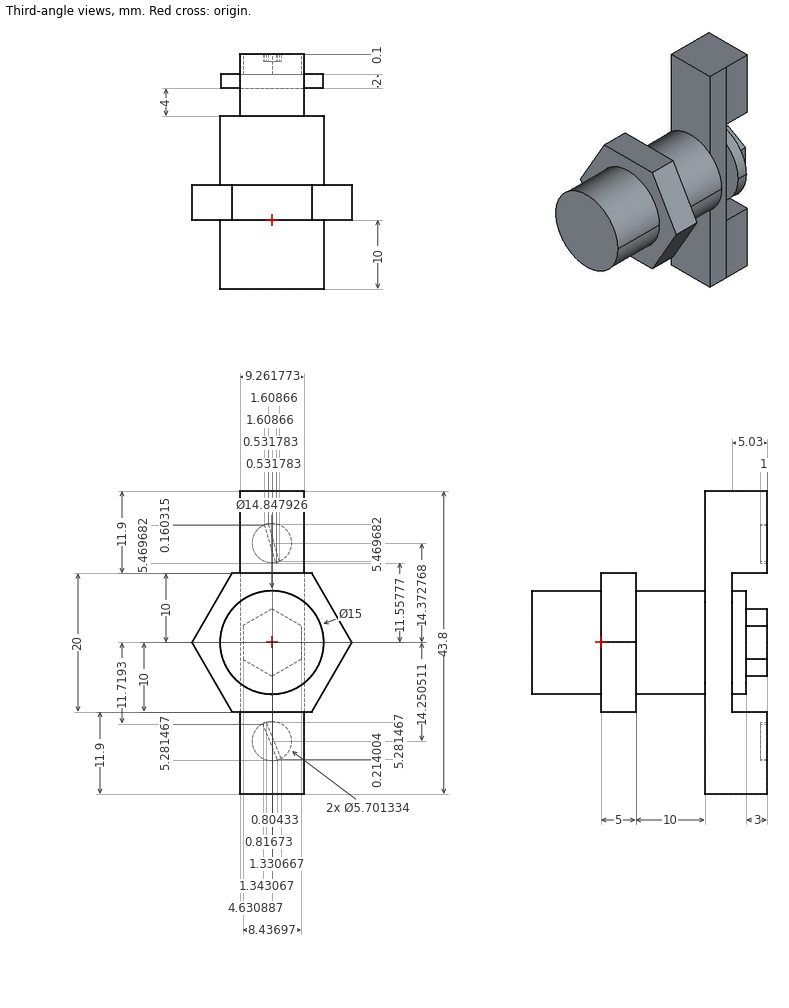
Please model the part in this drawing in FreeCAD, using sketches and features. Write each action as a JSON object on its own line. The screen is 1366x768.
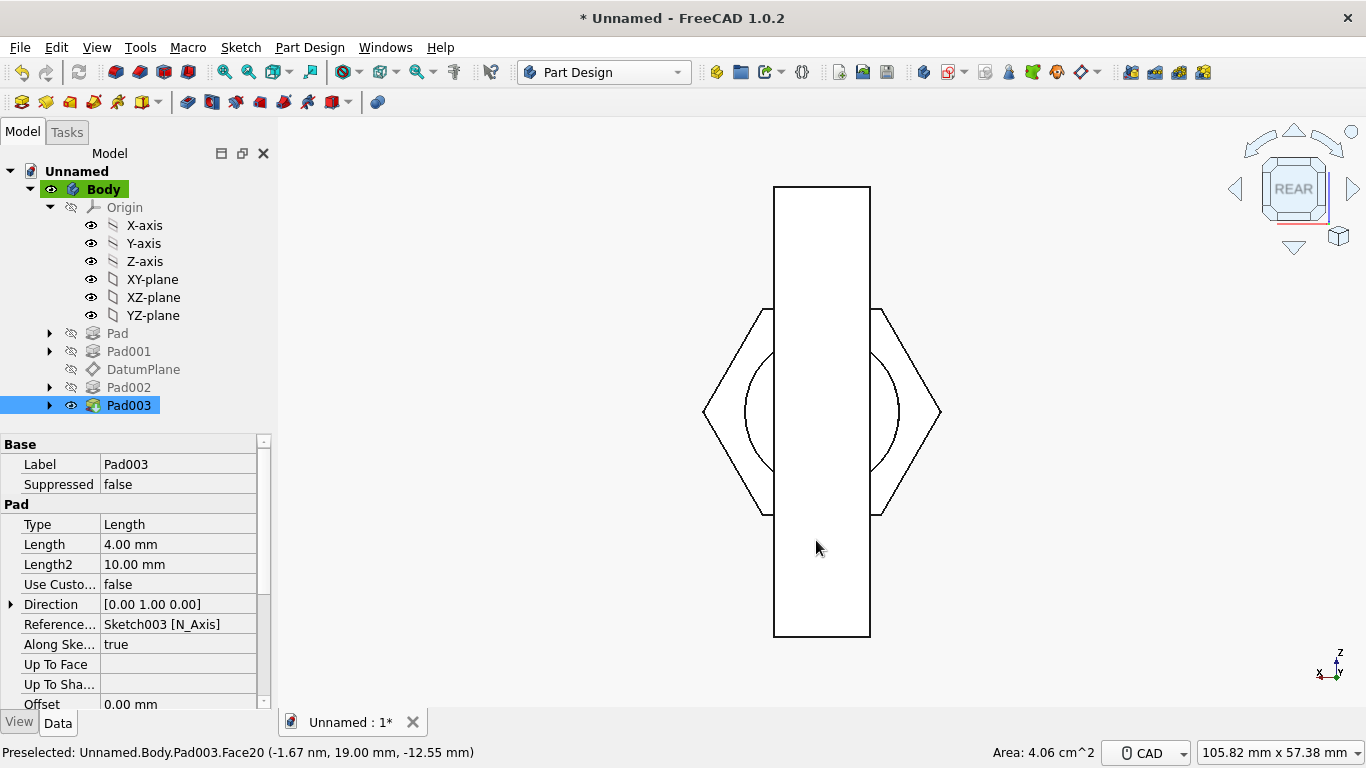
{"action": "left_click", "coordinate": [948, 72]}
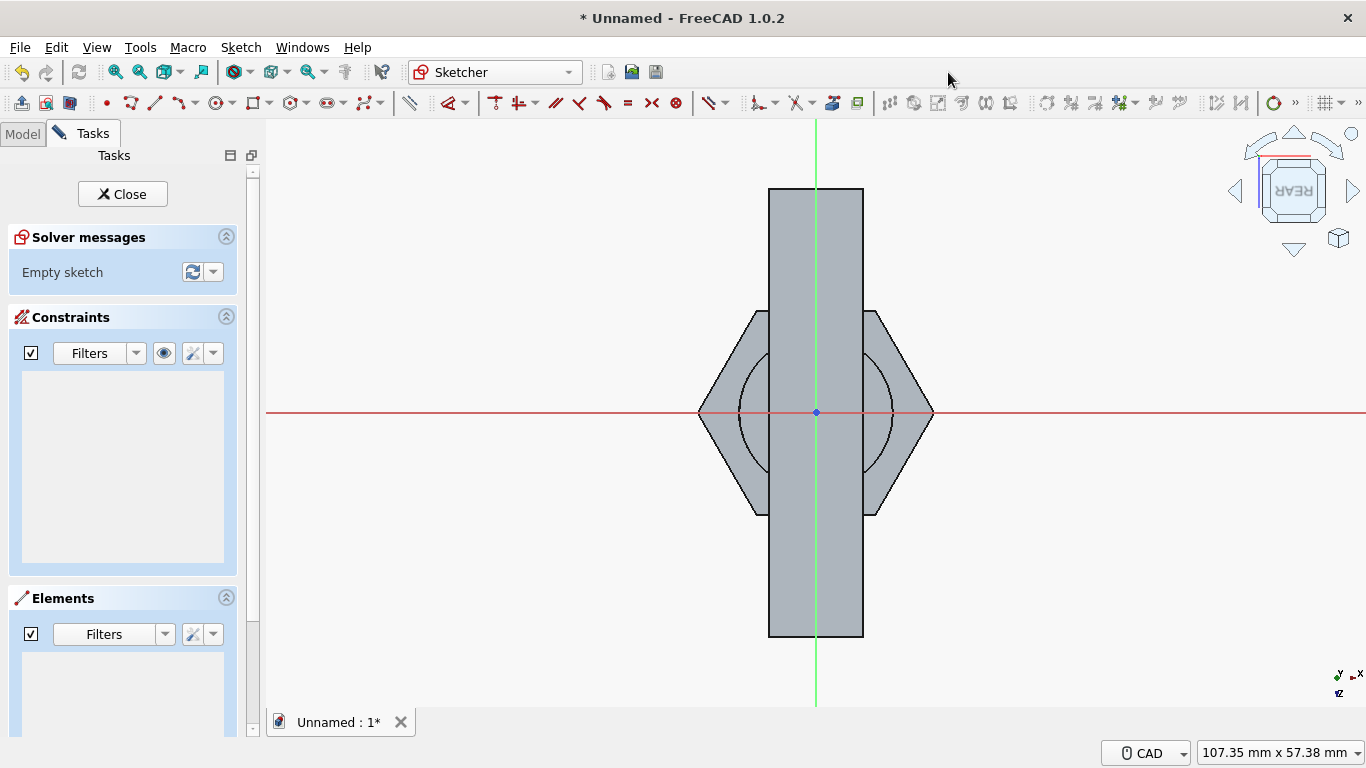
{"action": "left_click", "coordinate": [254, 104]}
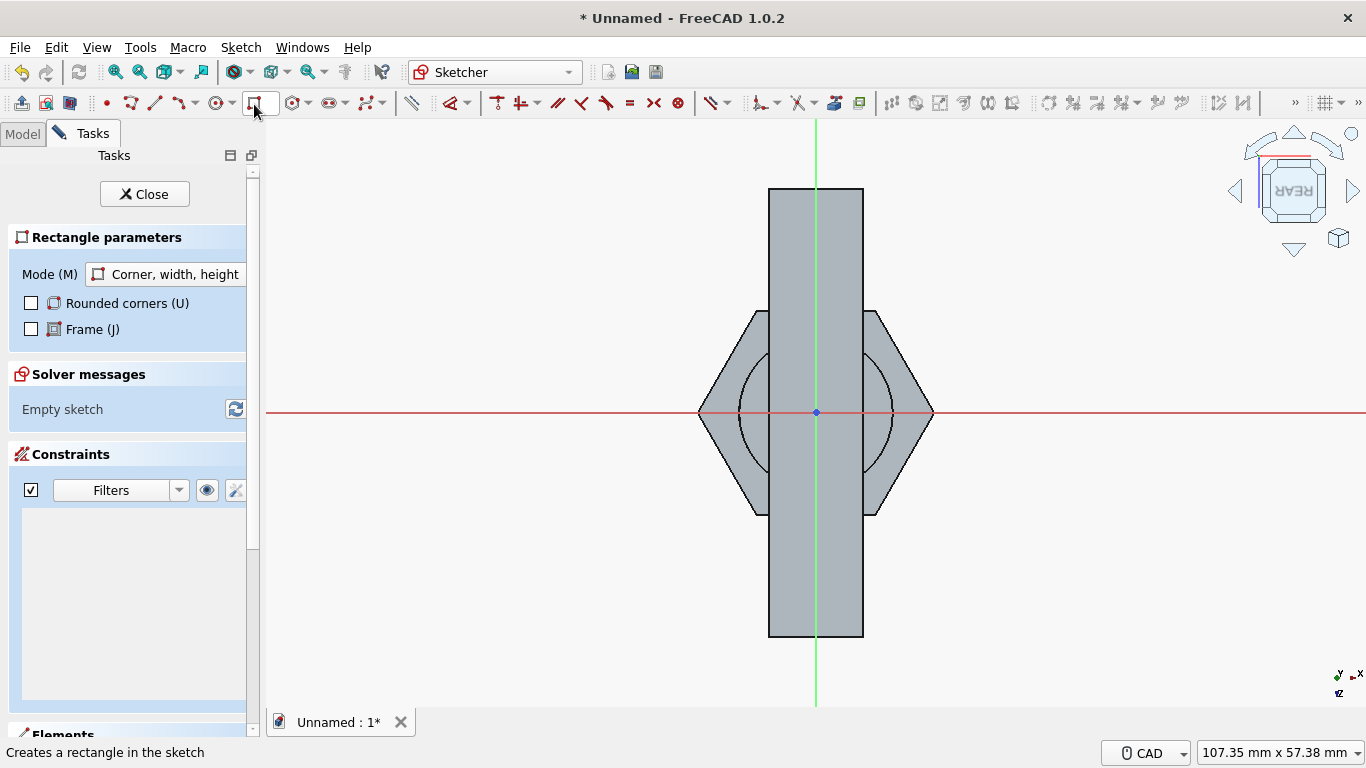
{"action": "left_click", "coordinate": [769, 189]}
{"action": "left_click", "coordinate": [863, 311]}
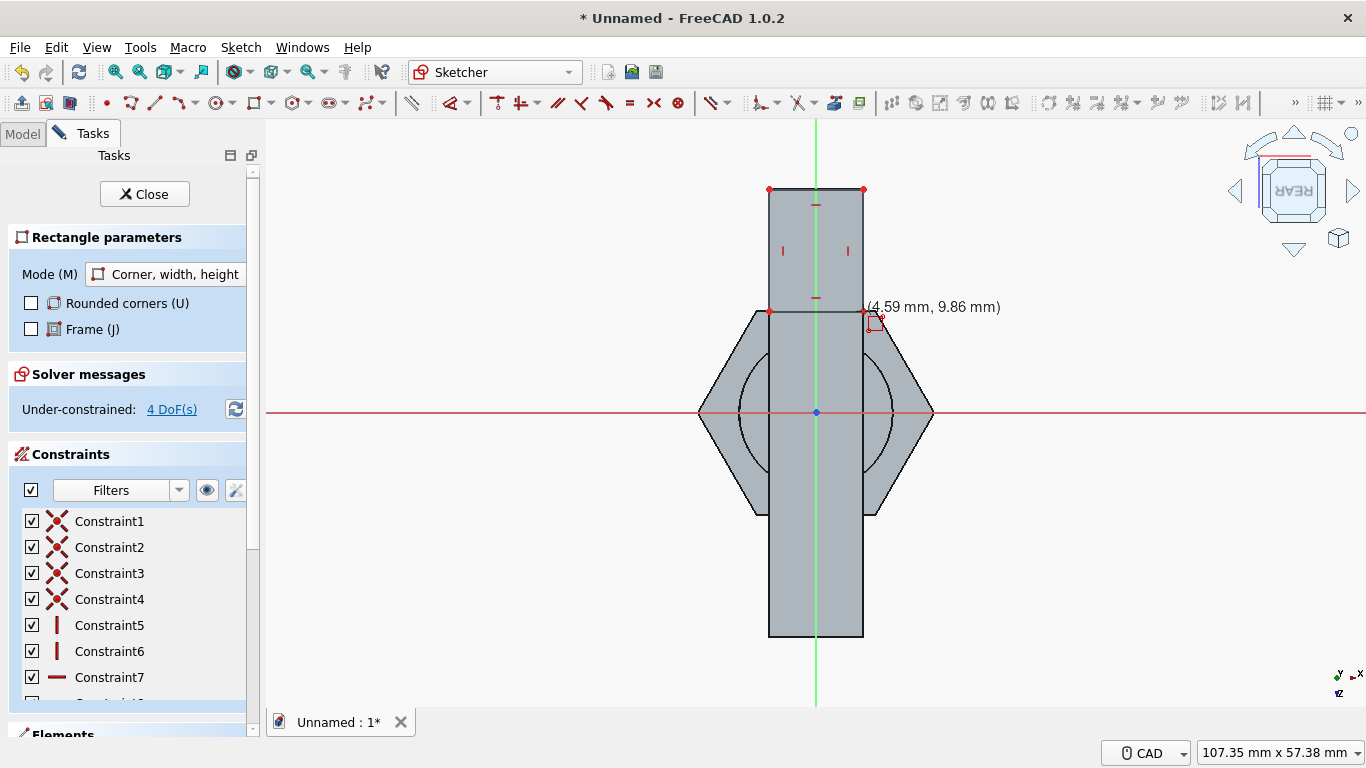
{"action": "left_click", "coordinate": [769, 515]}
{"action": "left_click", "coordinate": [863, 637]}
{"action": "key", "text": "Escape"}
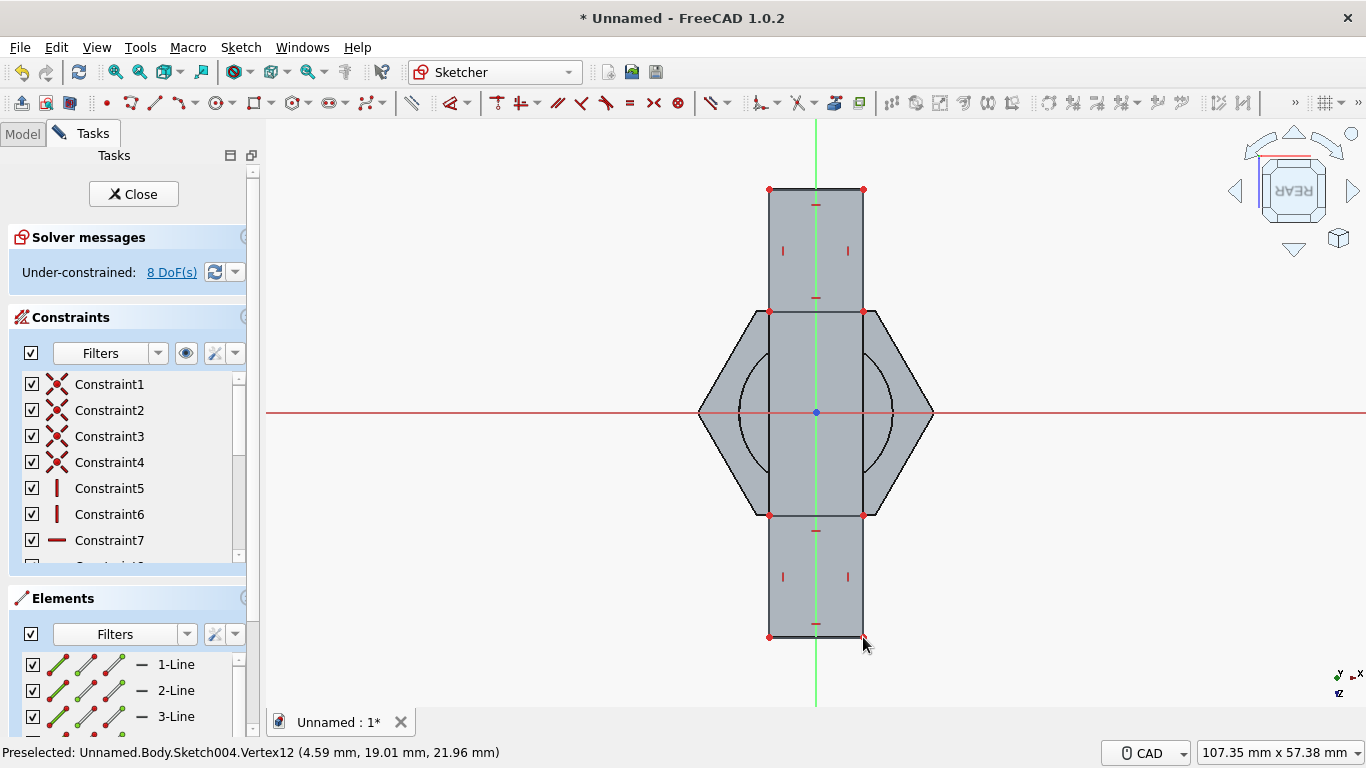
{"action": "left_click", "coordinate": [450, 104]}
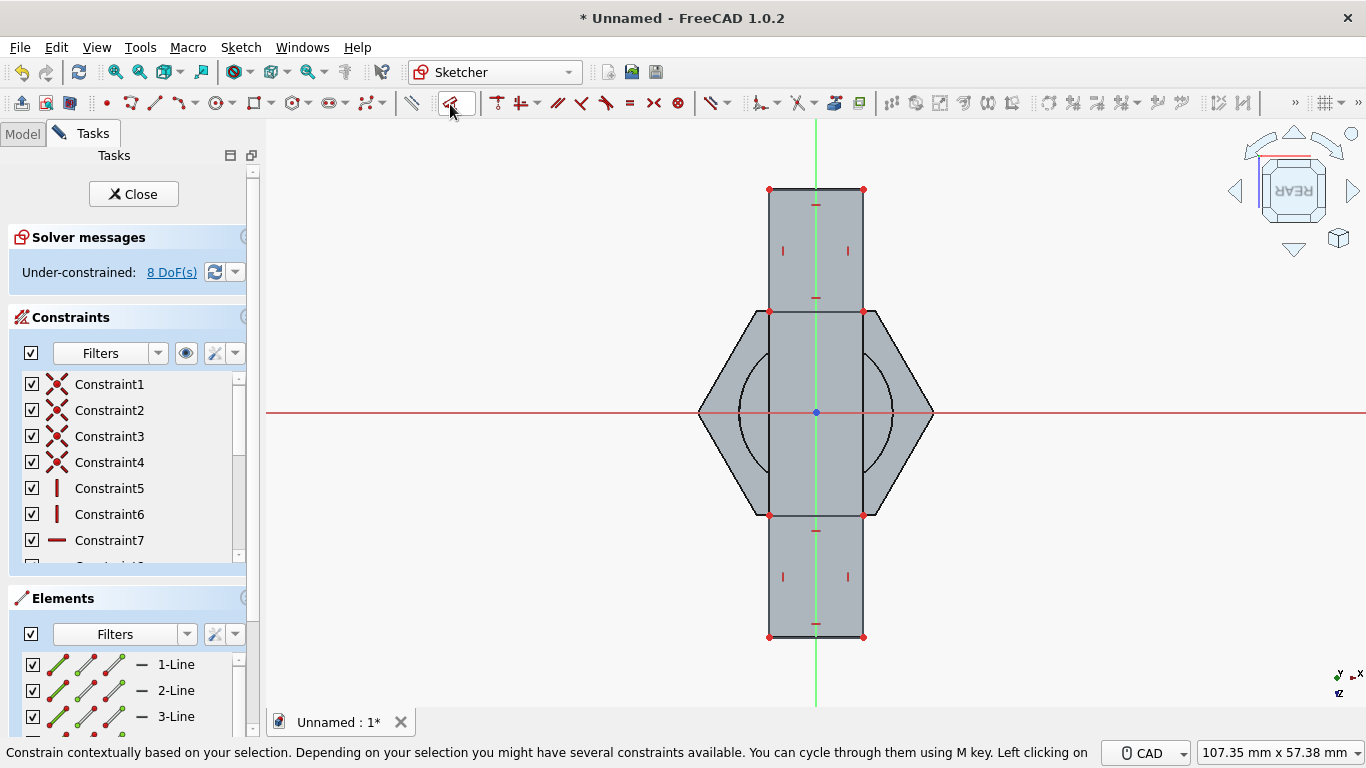
{"action": "left_click", "coordinate": [769, 312]}
{"action": "left_click", "coordinate": [735, 362]}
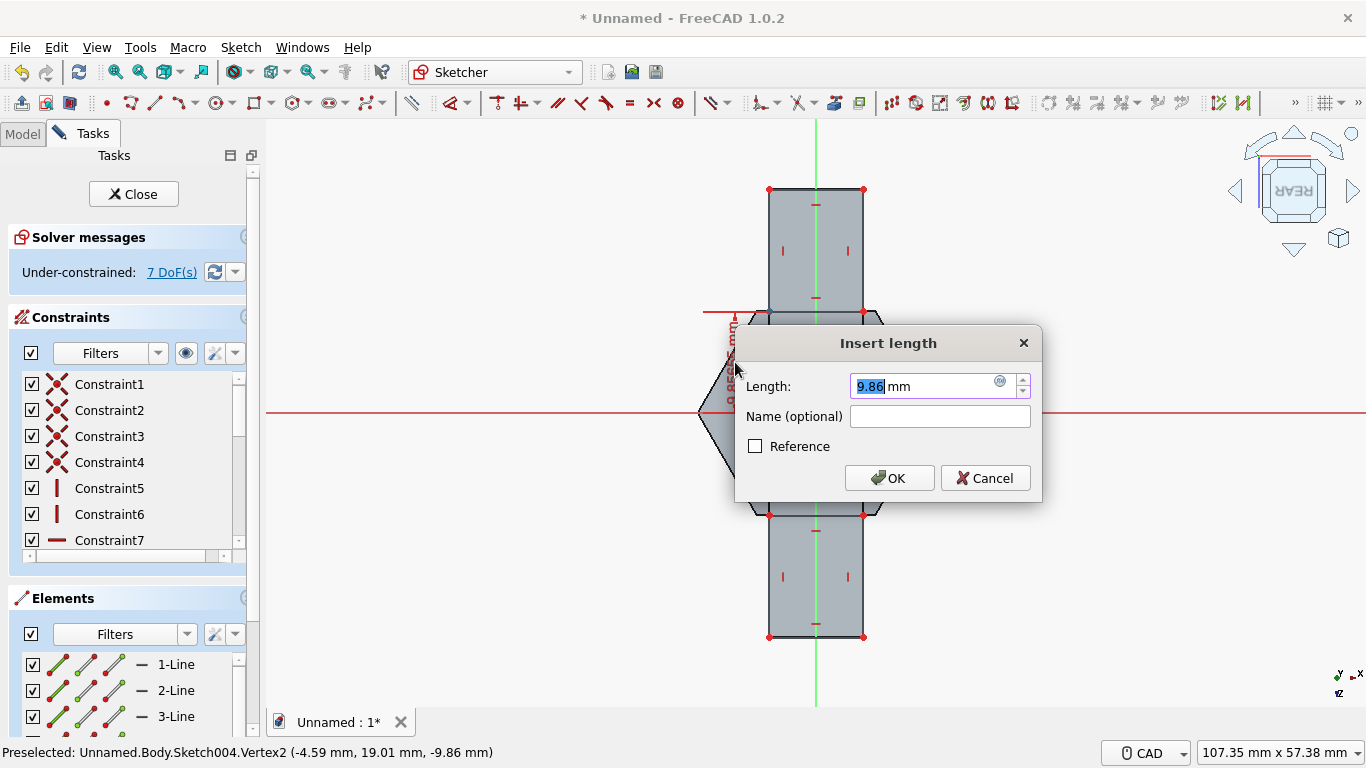
{"action": "type", "text": "10"}
{"action": "key", "text": "Return"}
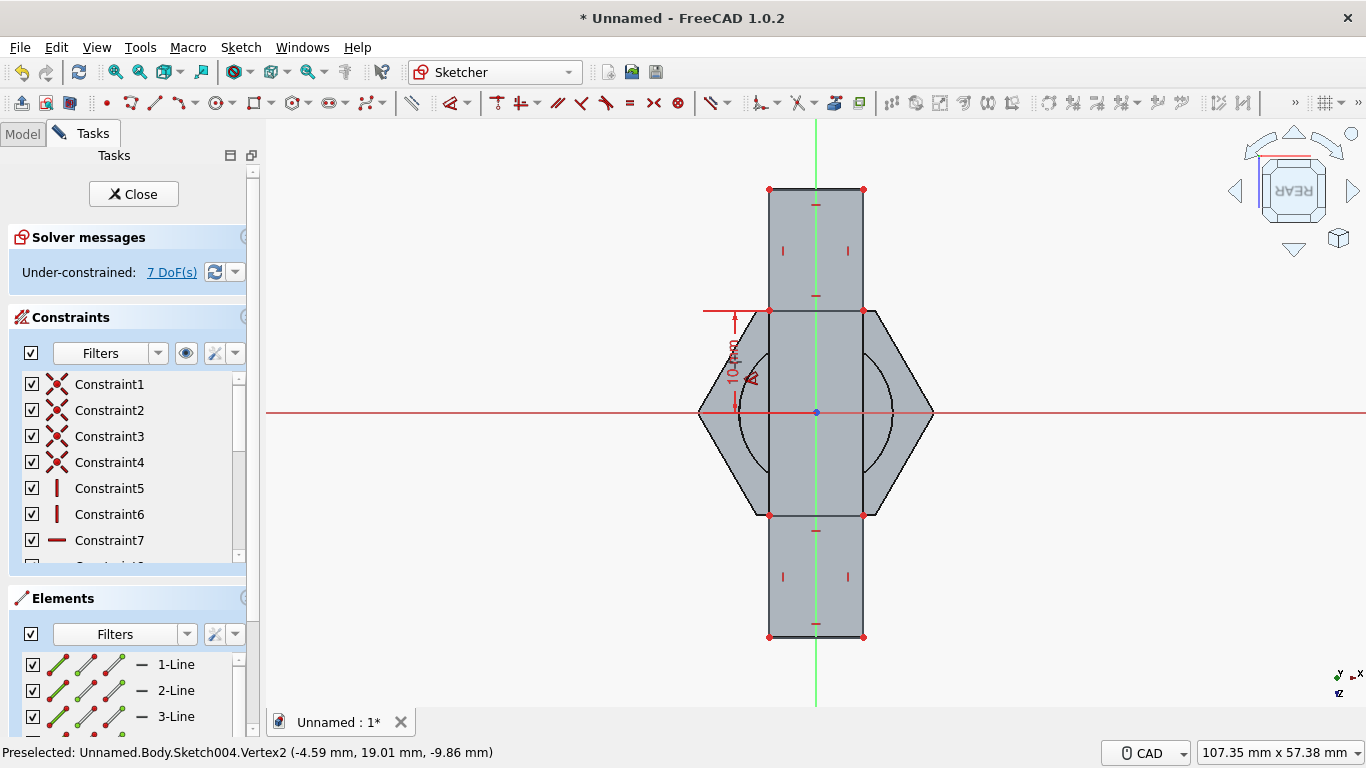
{"action": "left_click", "coordinate": [769, 516]}
{"action": "left_click", "coordinate": [735, 464]}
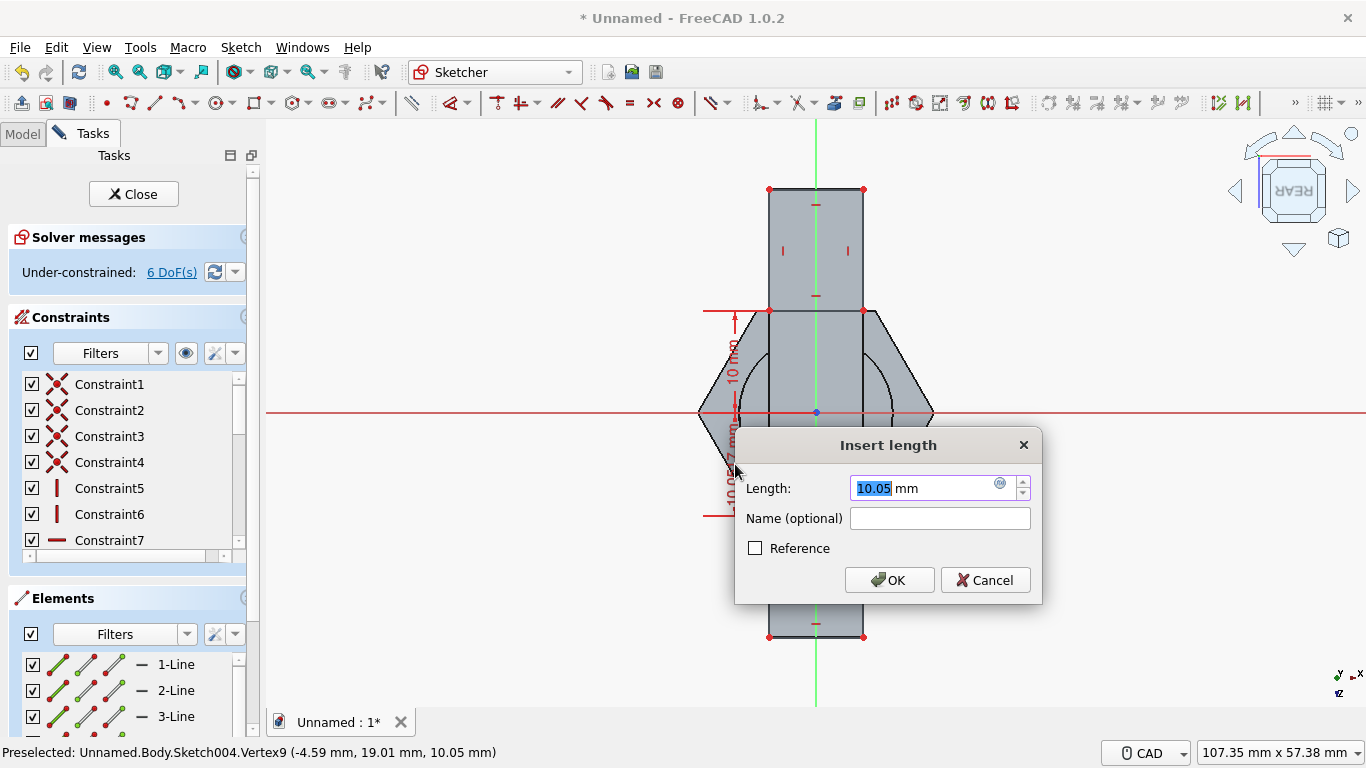
{"action": "type", "text": "10"}
{"action": "key", "text": "Return"}